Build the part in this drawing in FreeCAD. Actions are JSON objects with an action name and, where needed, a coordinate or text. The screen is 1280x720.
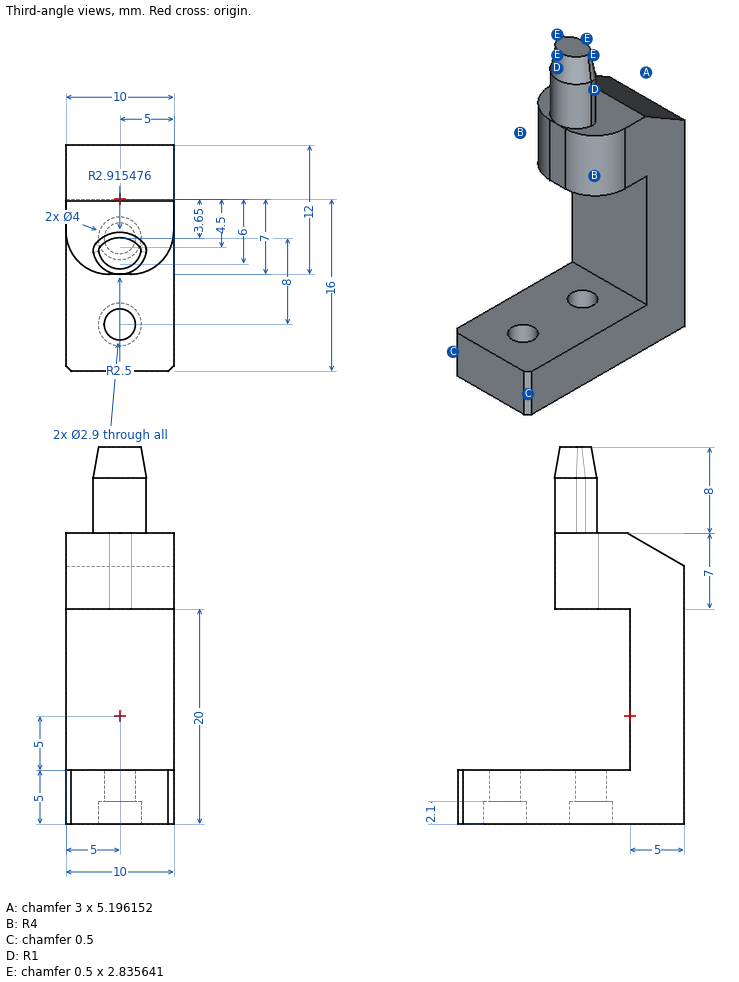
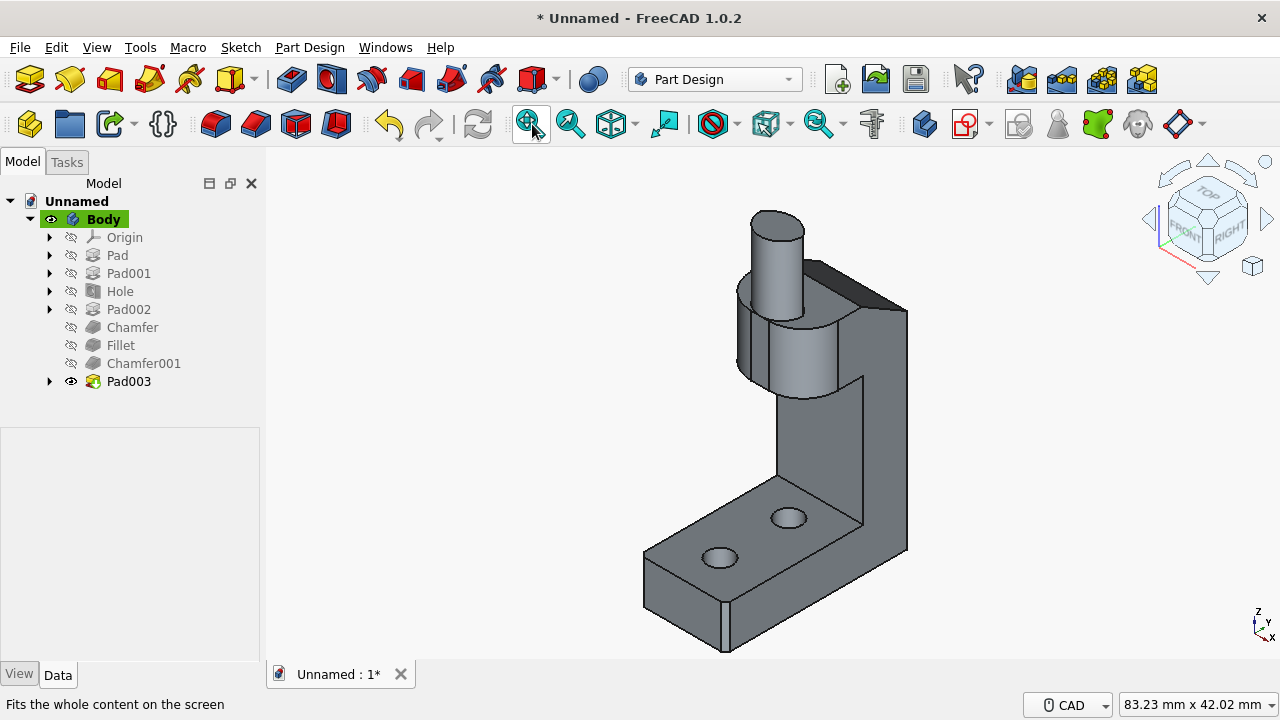
{"action": "key", "text": "2"}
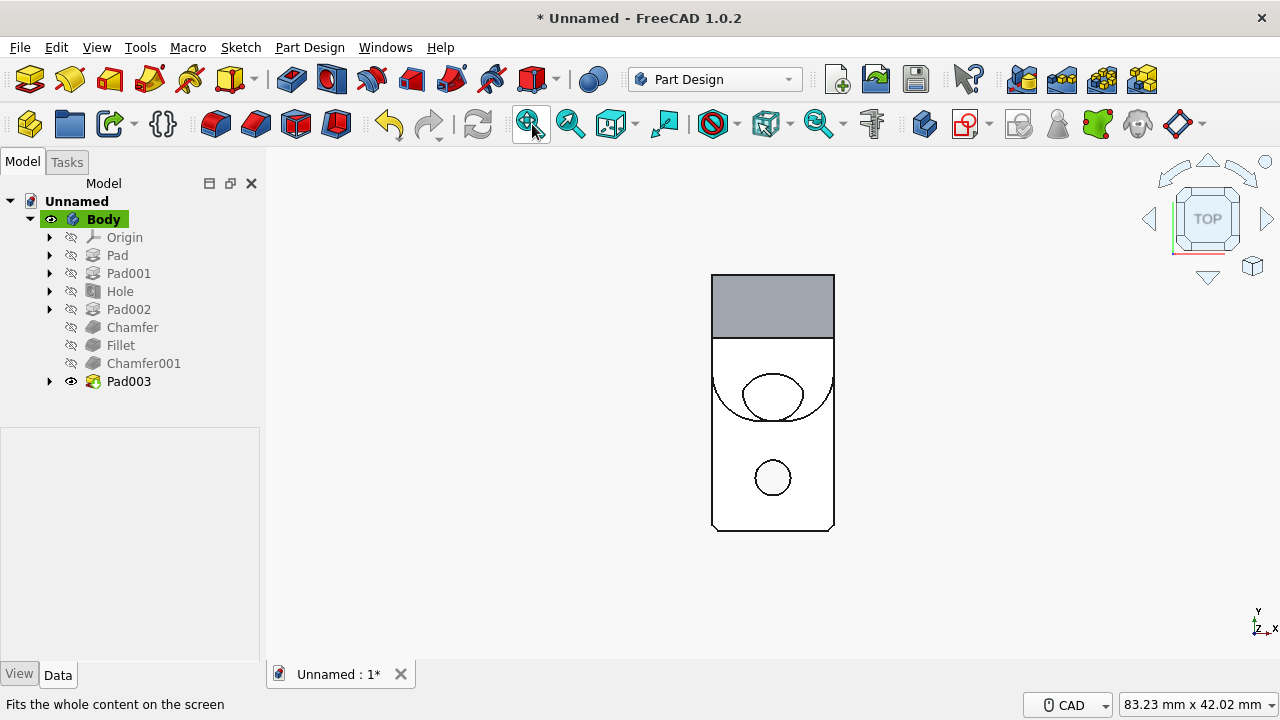
{"action": "key", "text": "0"}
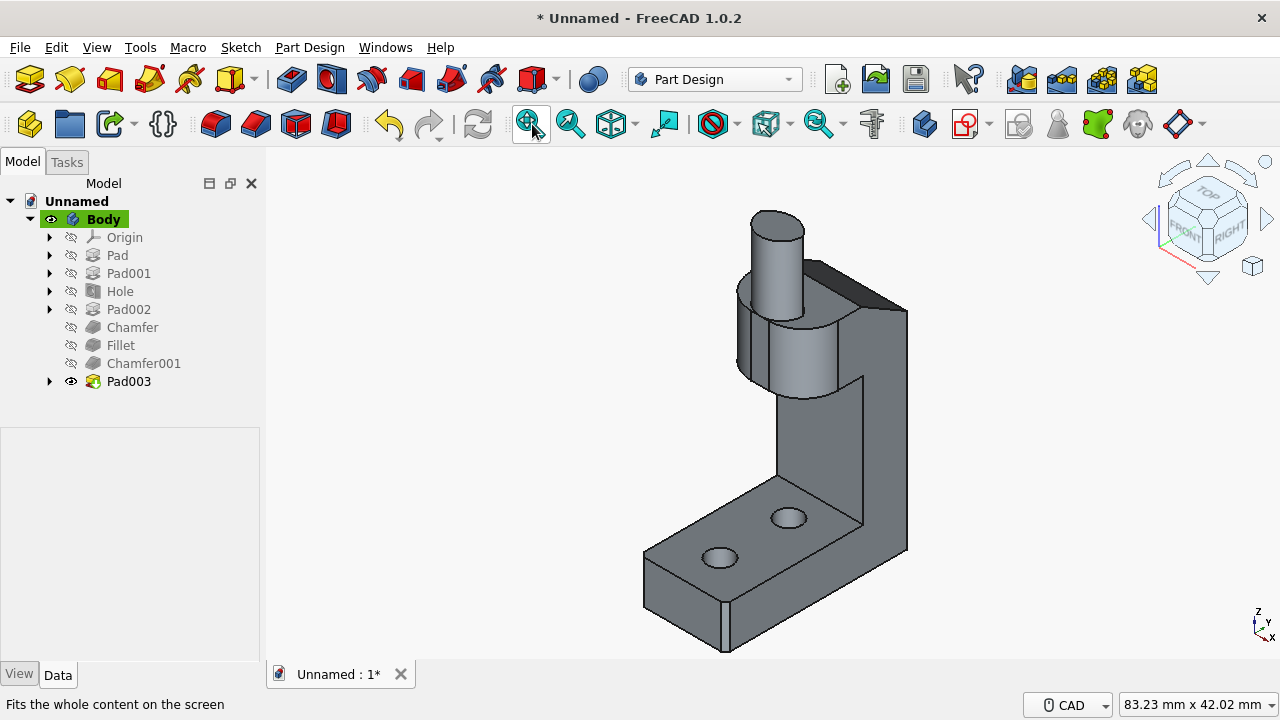
{"action": "key", "text": "1"}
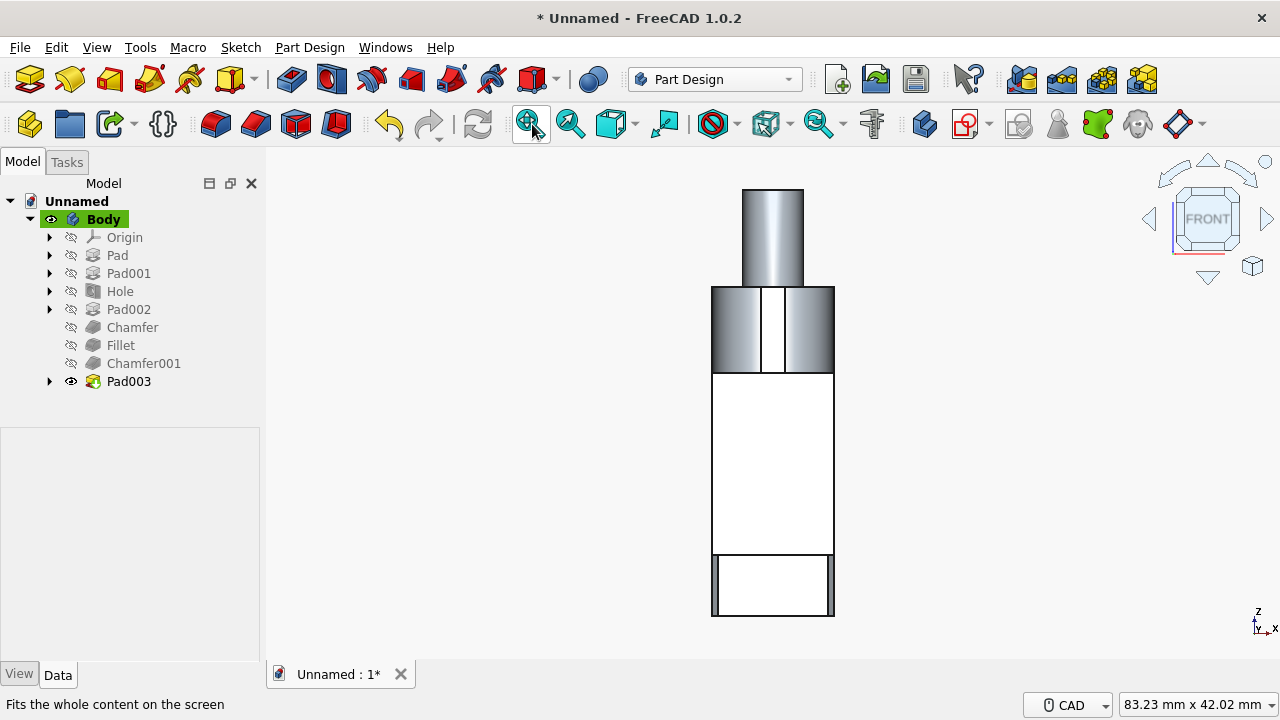
{"action": "key", "text": "3"}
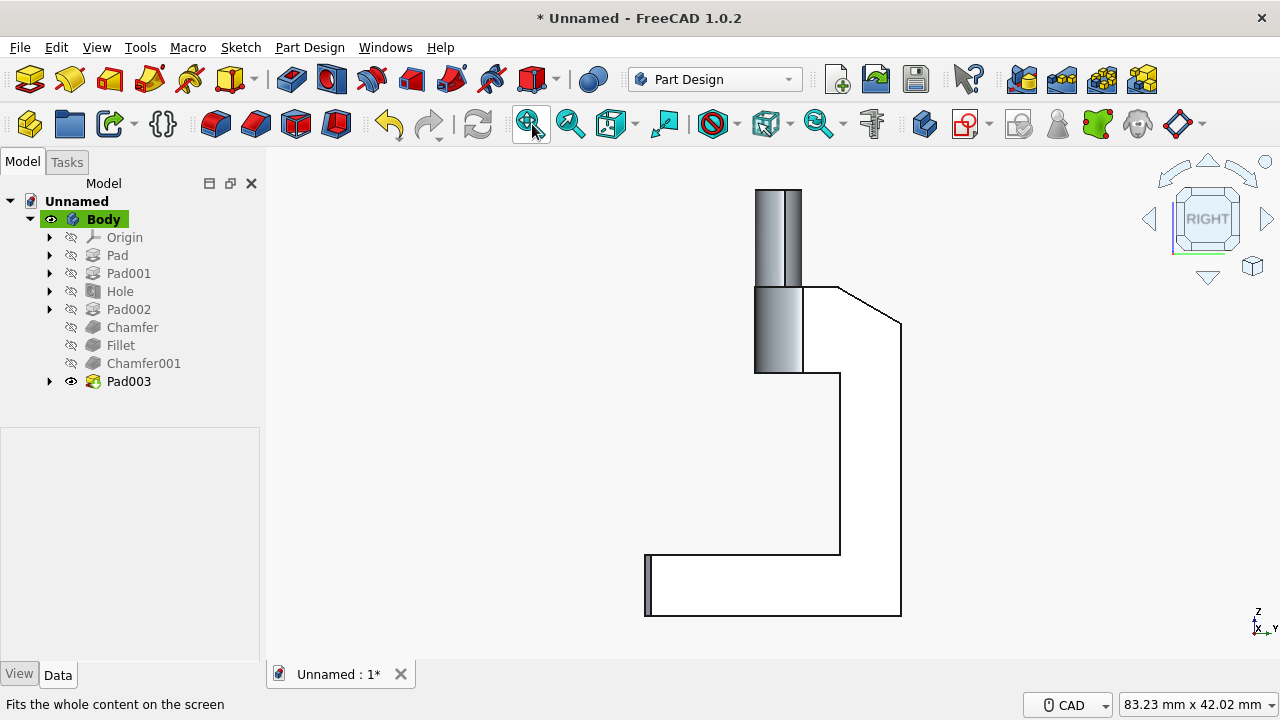
{"action": "left_click", "coordinate": [785, 238]}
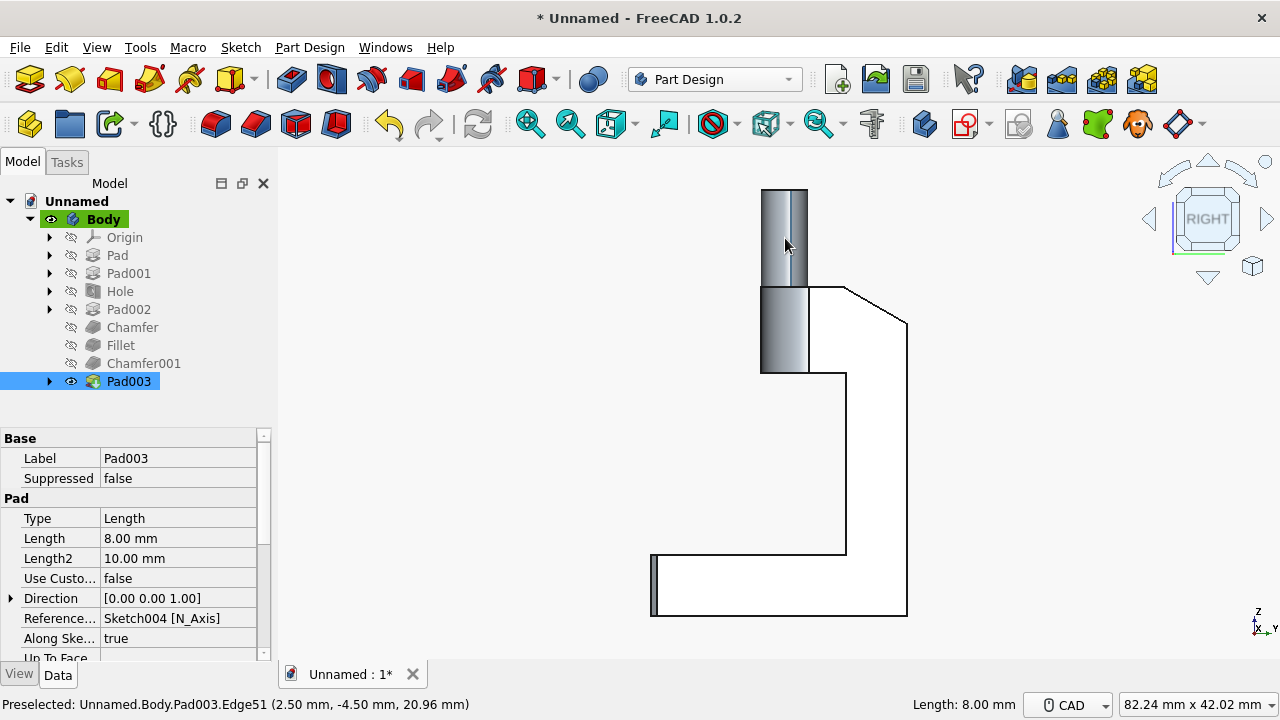
{"action": "key", "text": "5"}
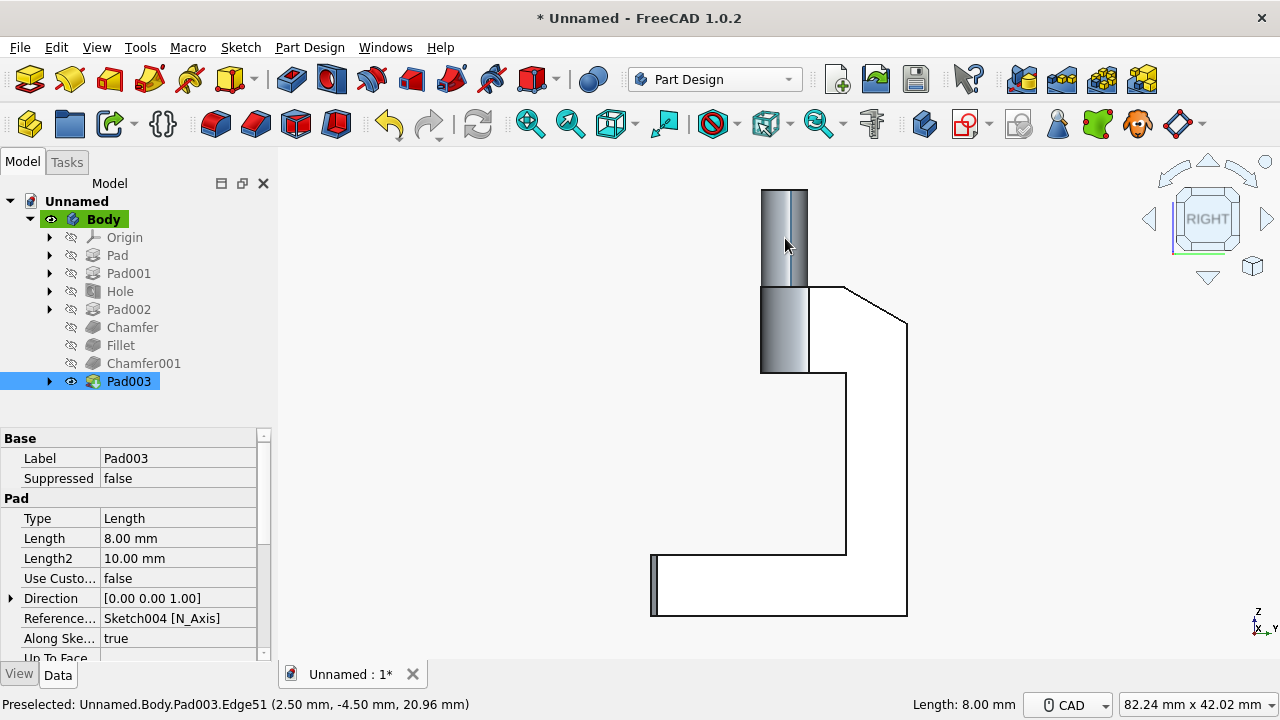
{"action": "key", "text": "4"}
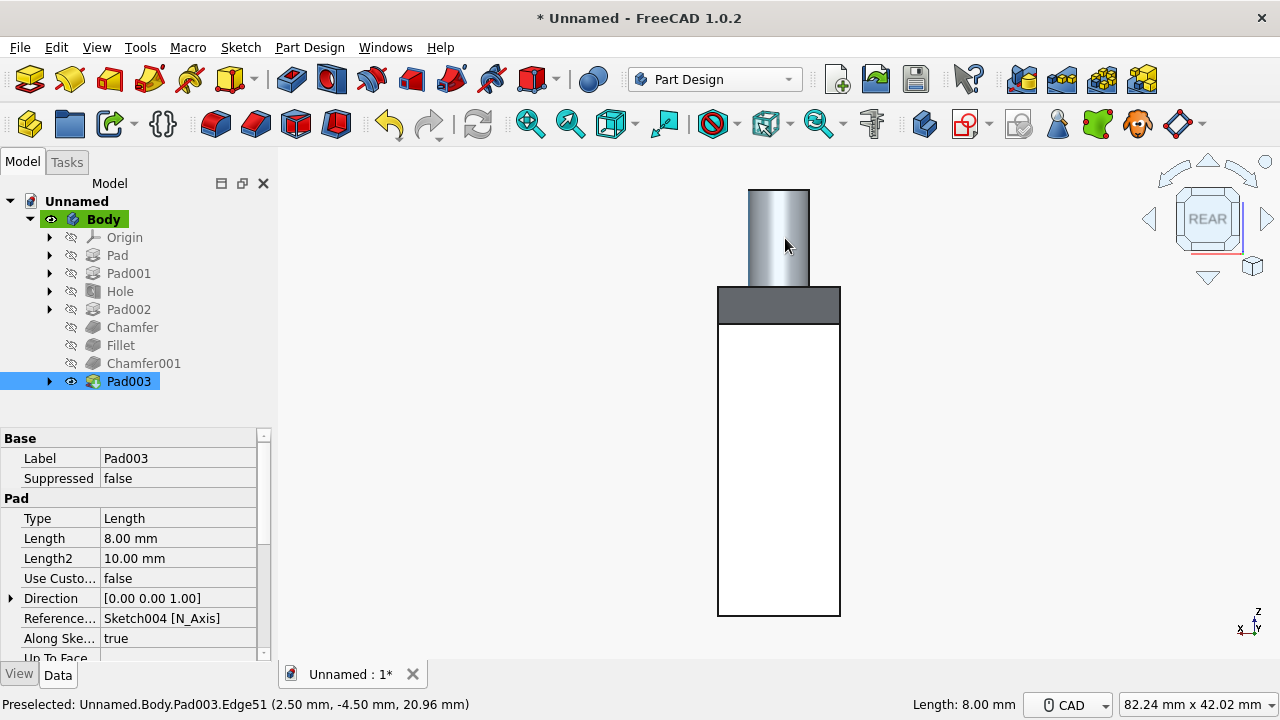
{"action": "key", "text": "6"}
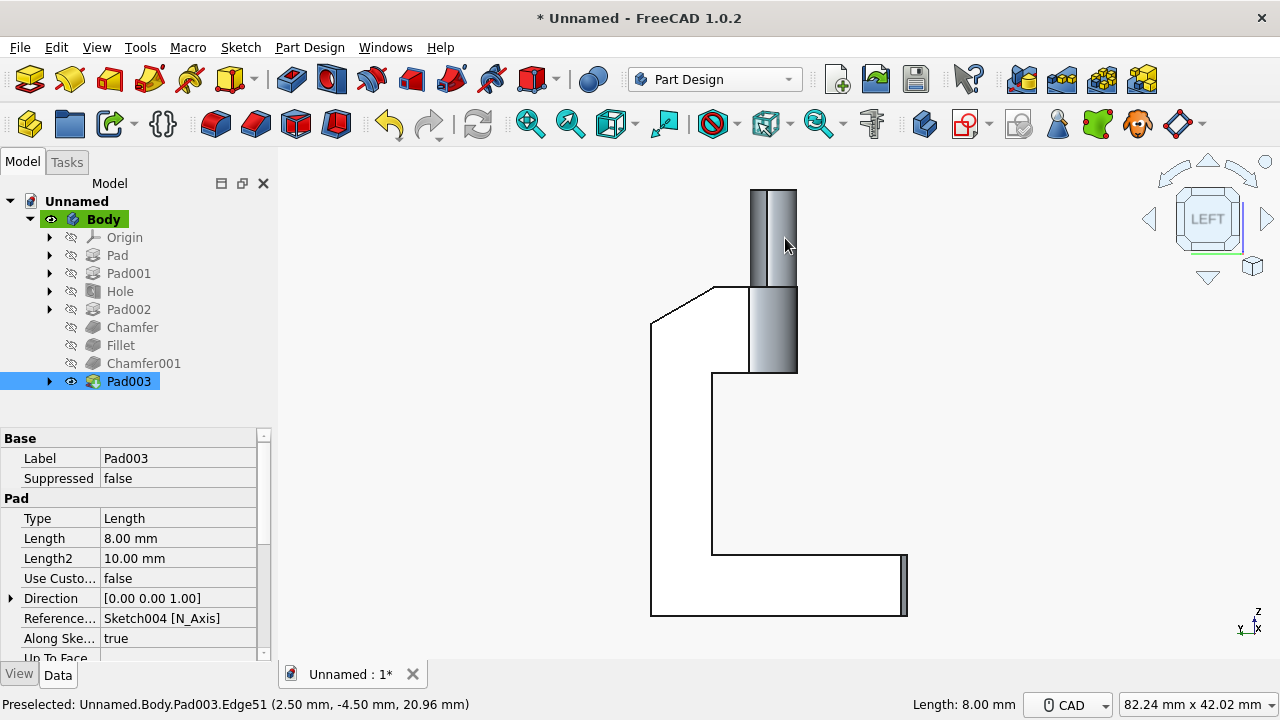
{"action": "left_click", "coordinate": [767, 238], "text": "ctrl"}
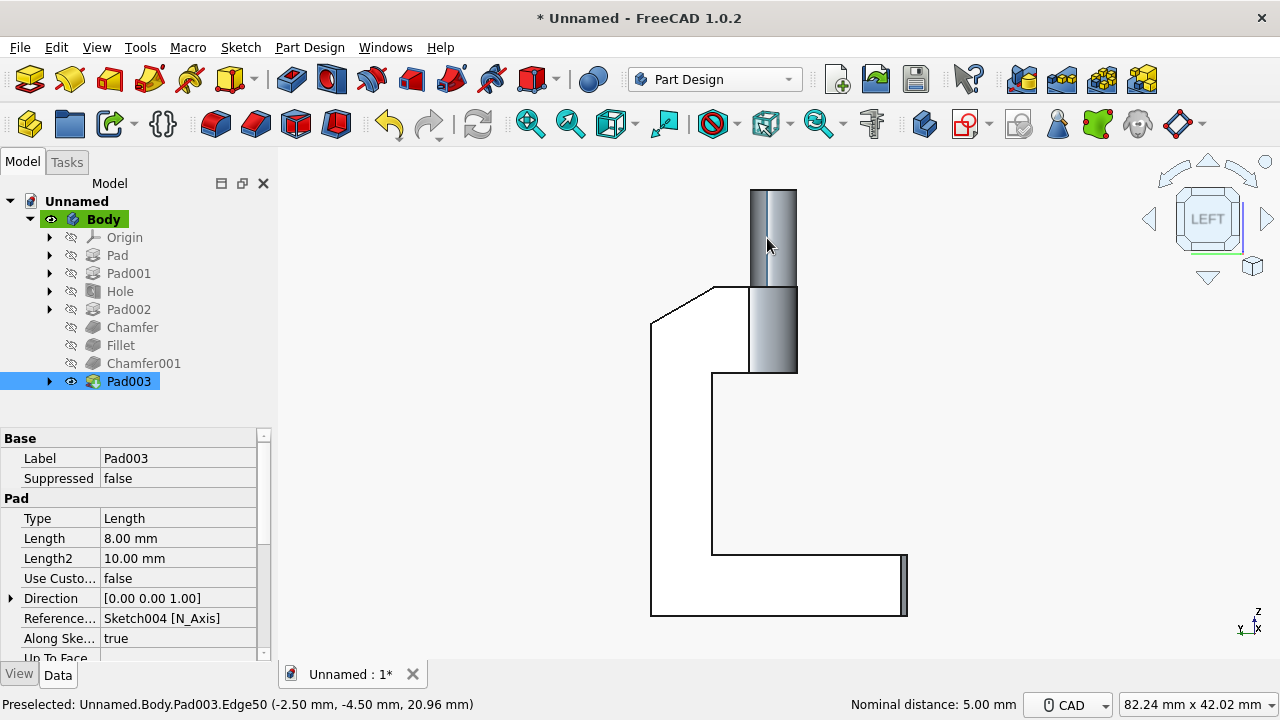
{"action": "left_click", "coordinate": [216, 124]}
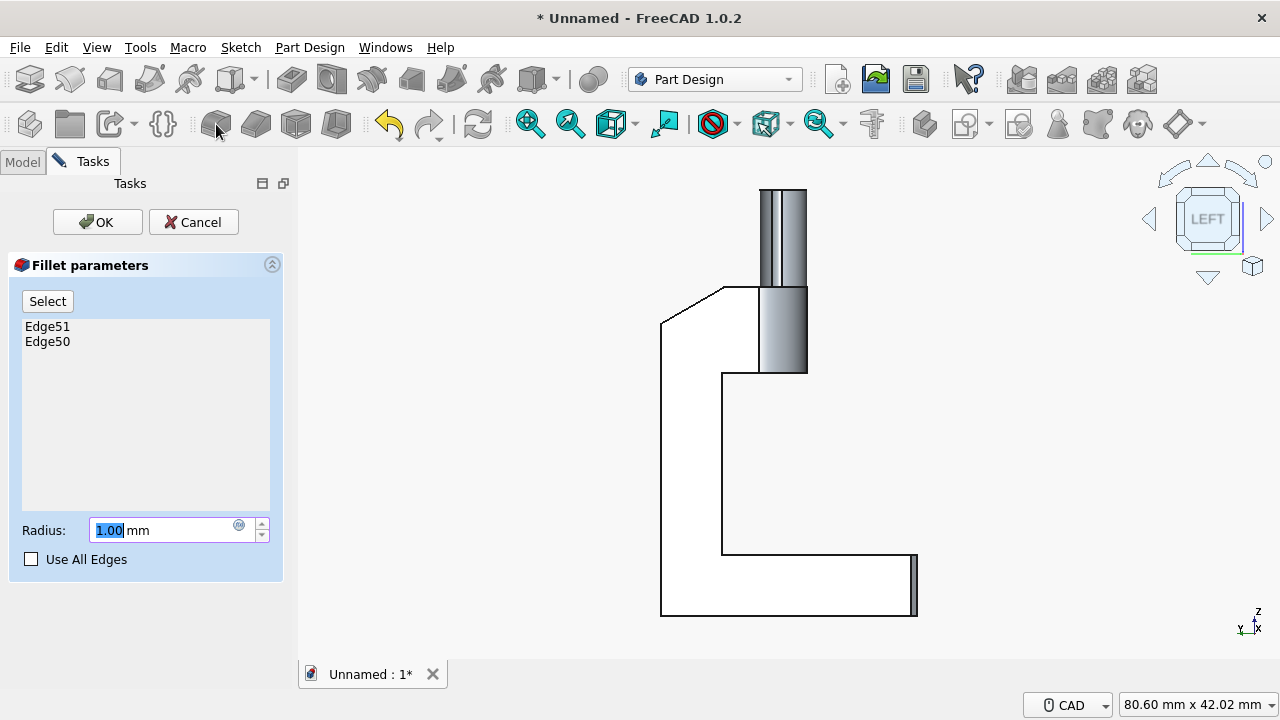
{"action": "type", "text": "1"}
{"action": "key", "text": "Tab"}